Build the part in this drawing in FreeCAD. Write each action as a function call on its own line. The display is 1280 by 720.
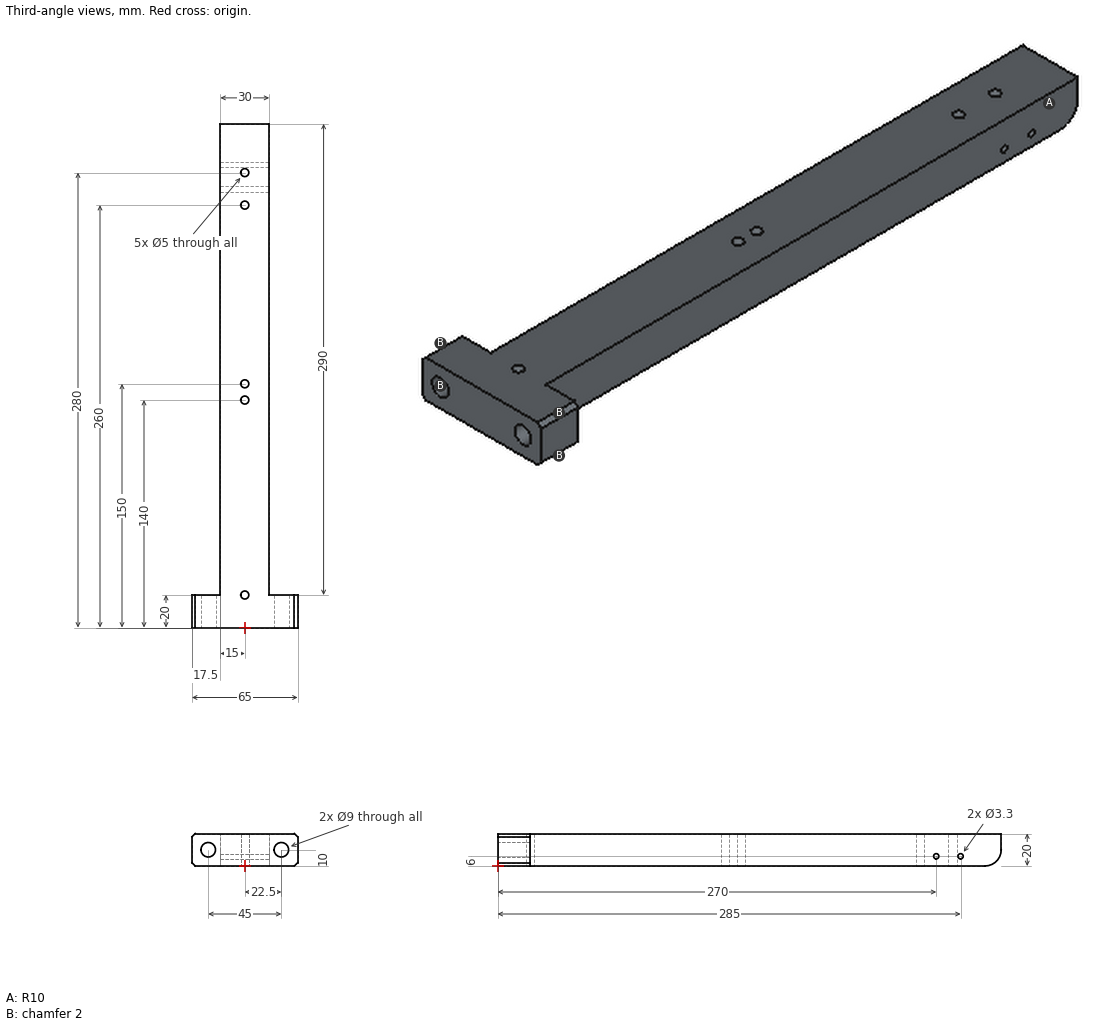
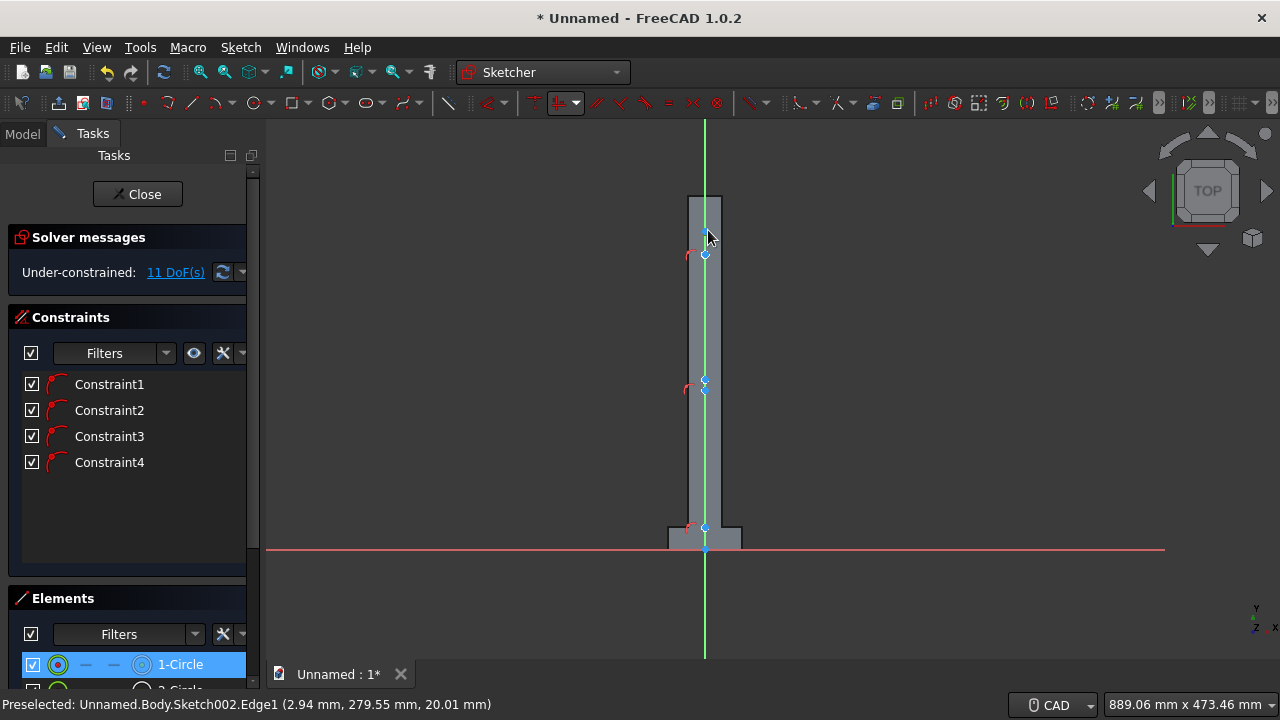
scroll(707, 378, up, 10)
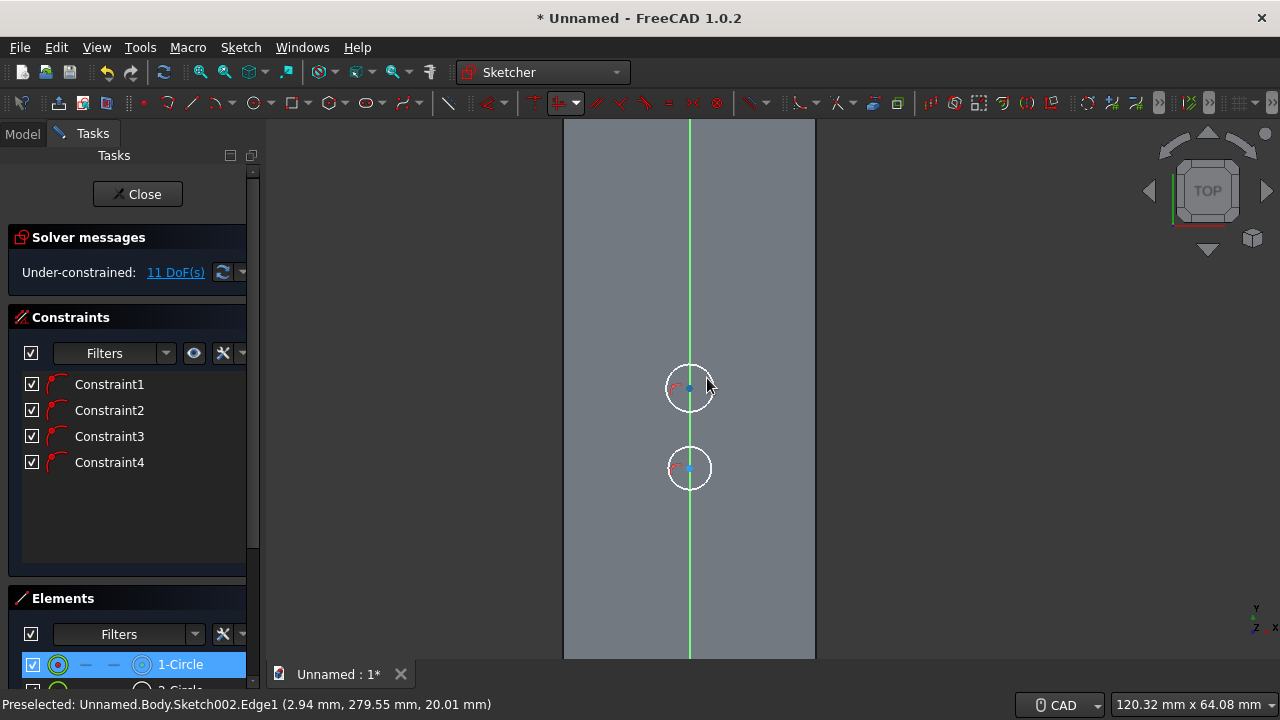
click(707, 371)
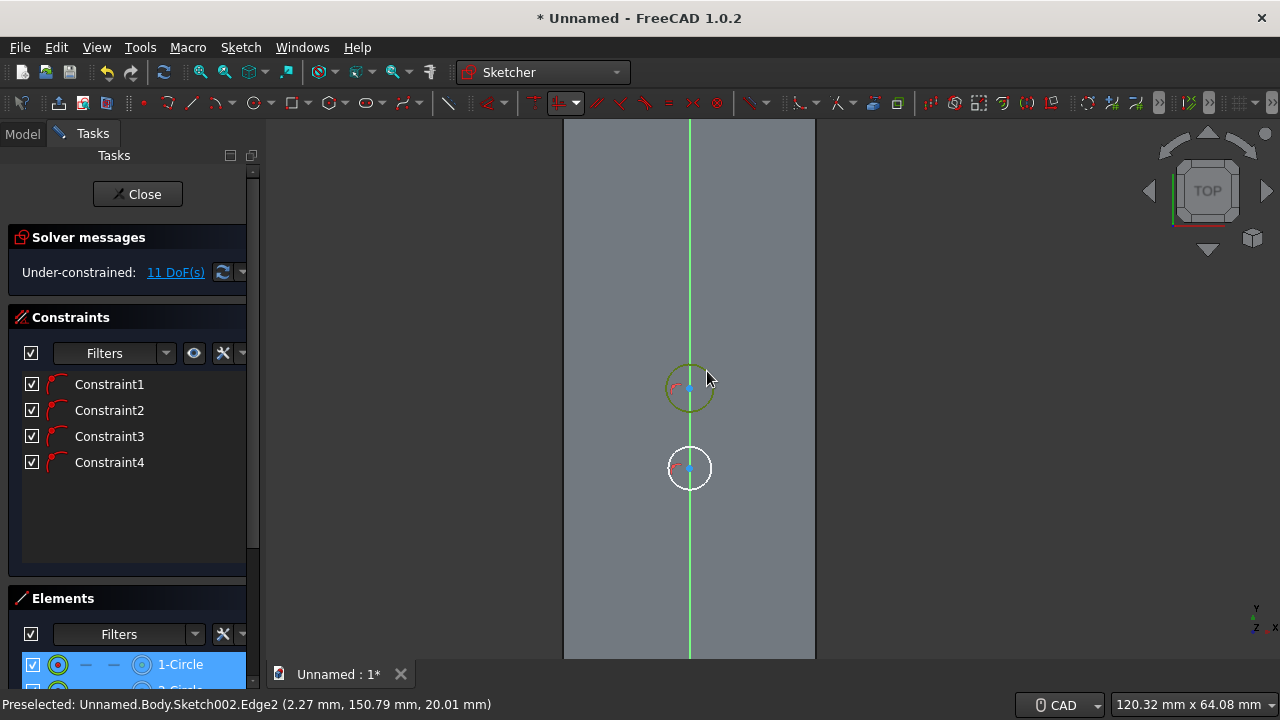
scroll(707, 379, down, 10)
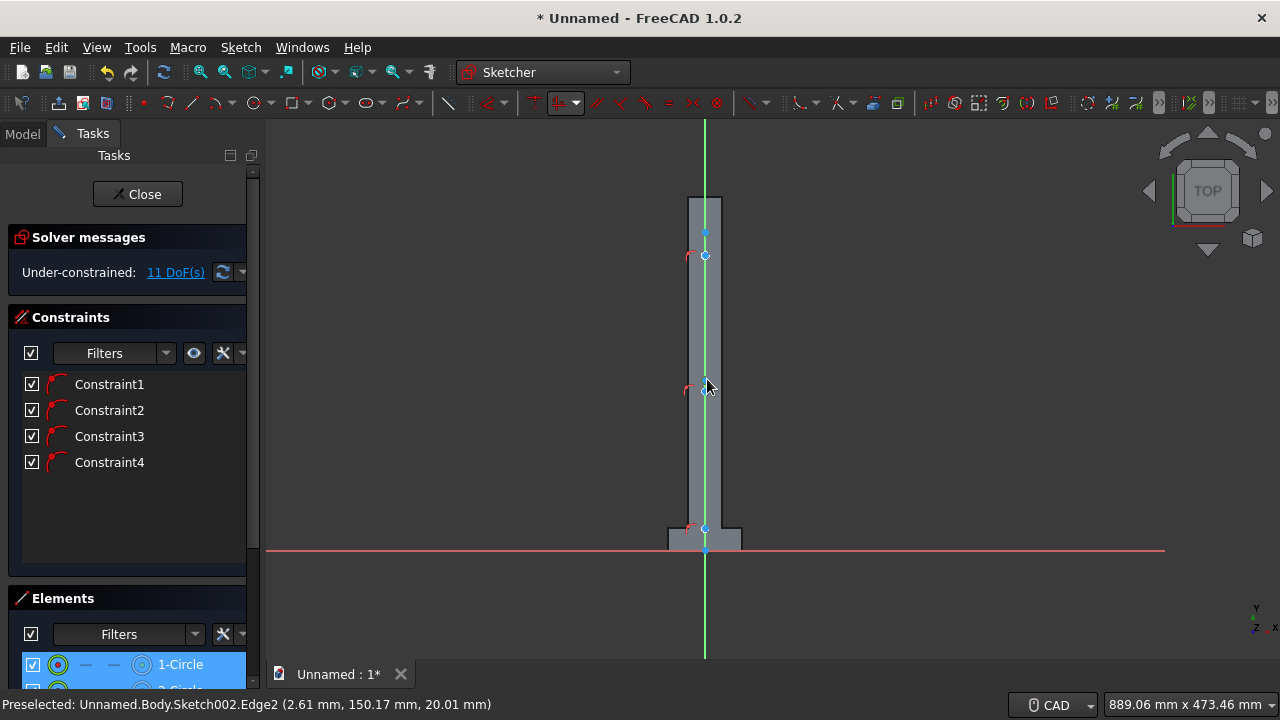
scroll(707, 527, up, 10)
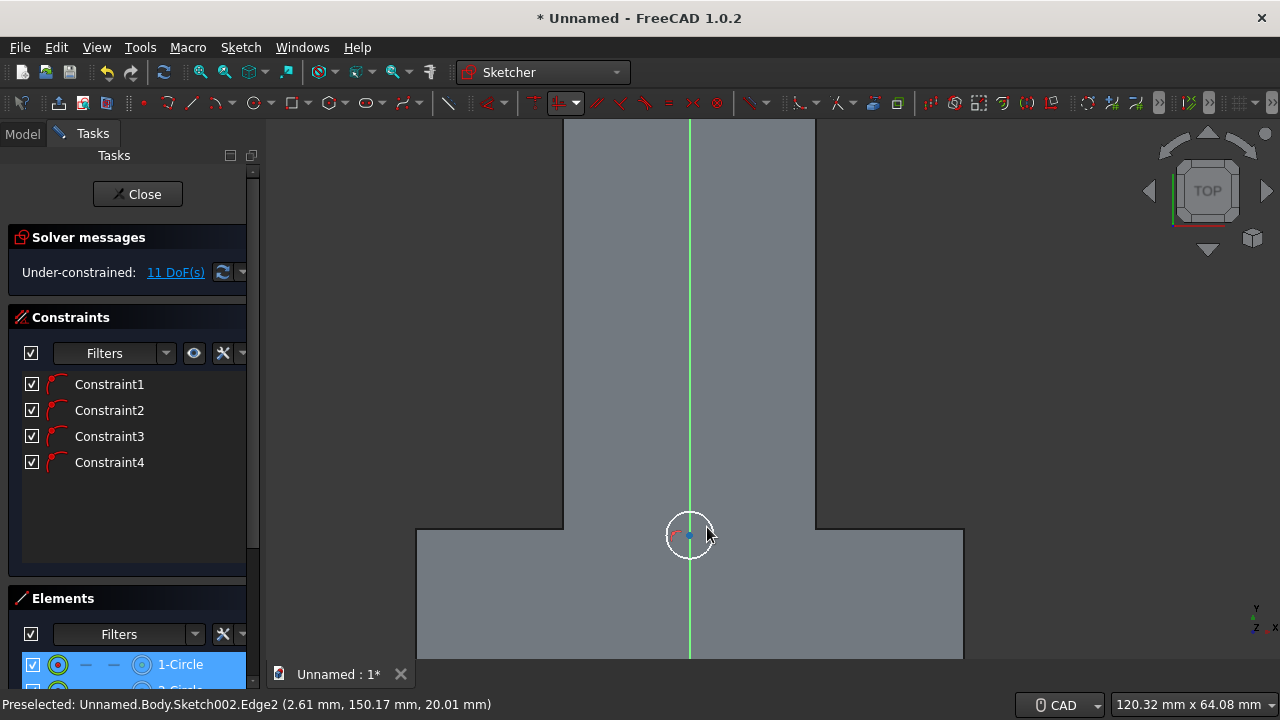
click(706, 519)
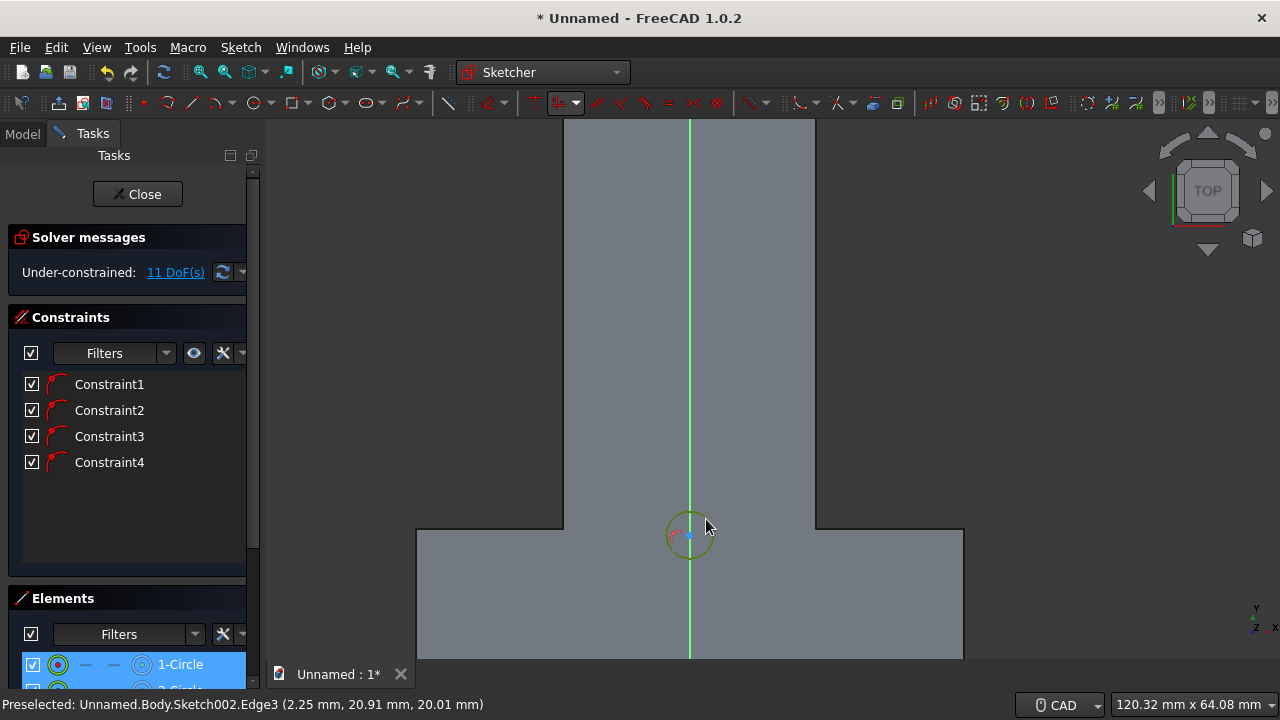
scroll(707, 527, down, 10)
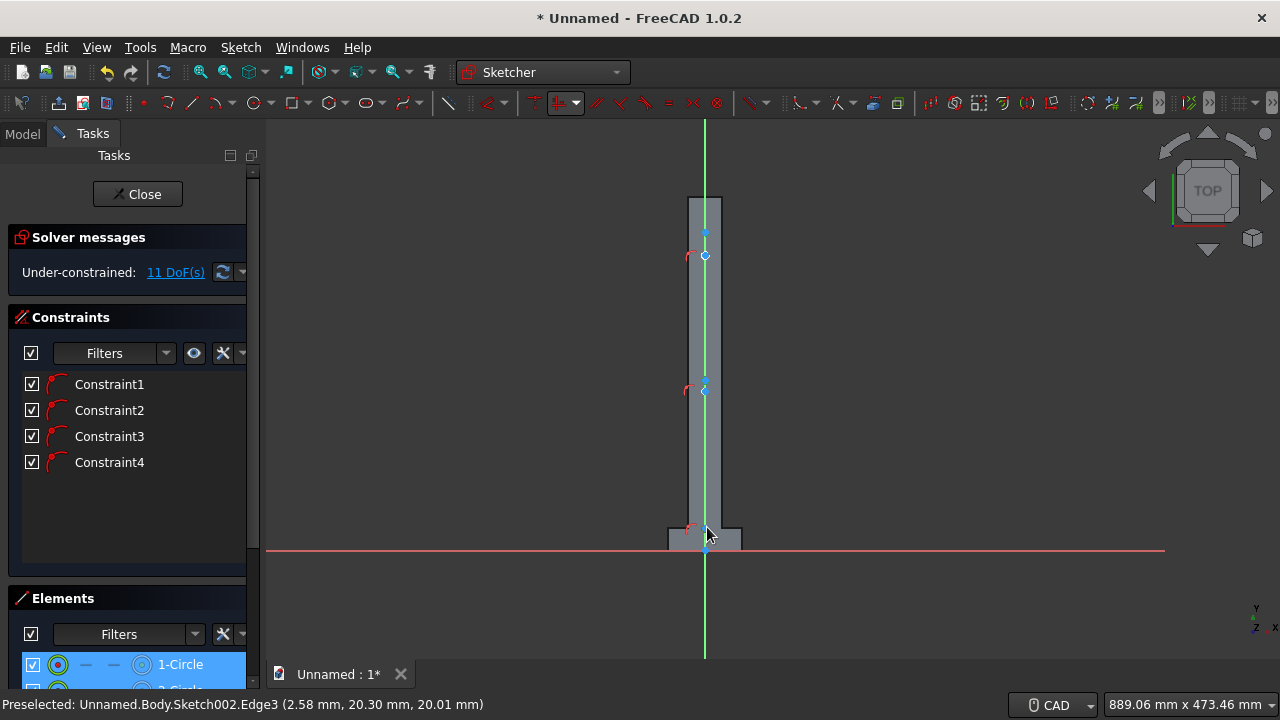
scroll(708, 253, up, 9)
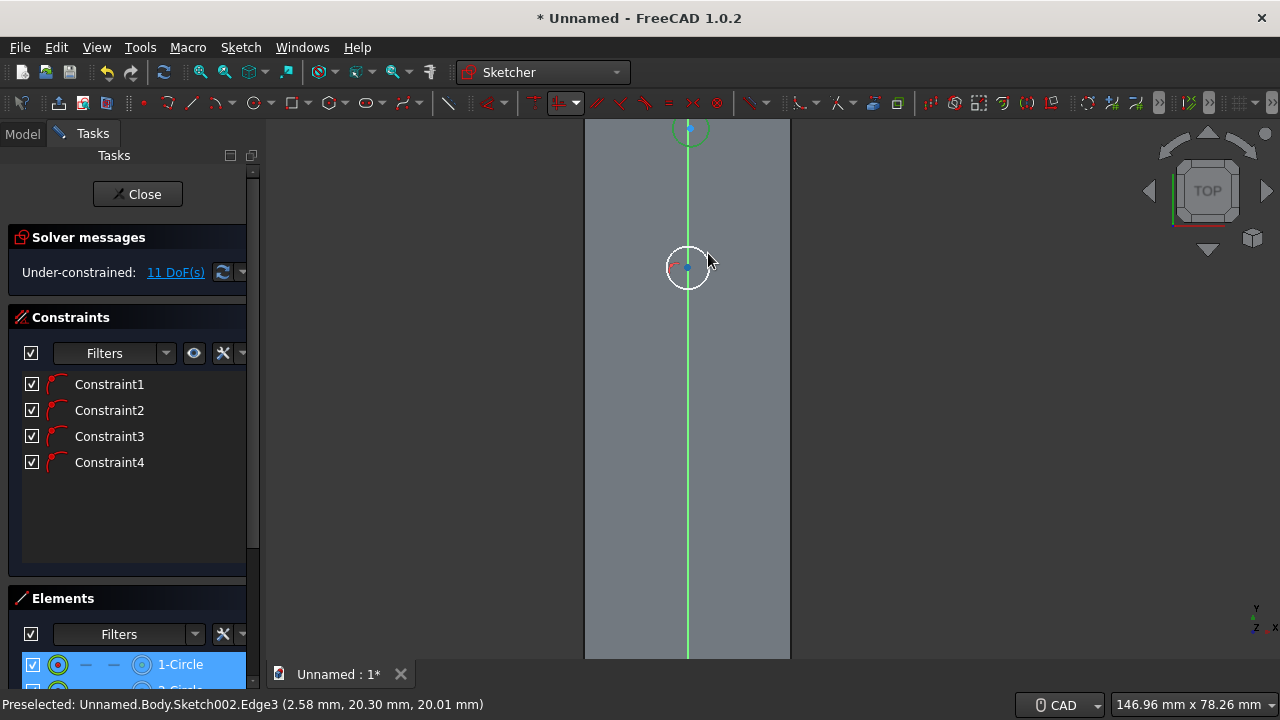
click(703, 253)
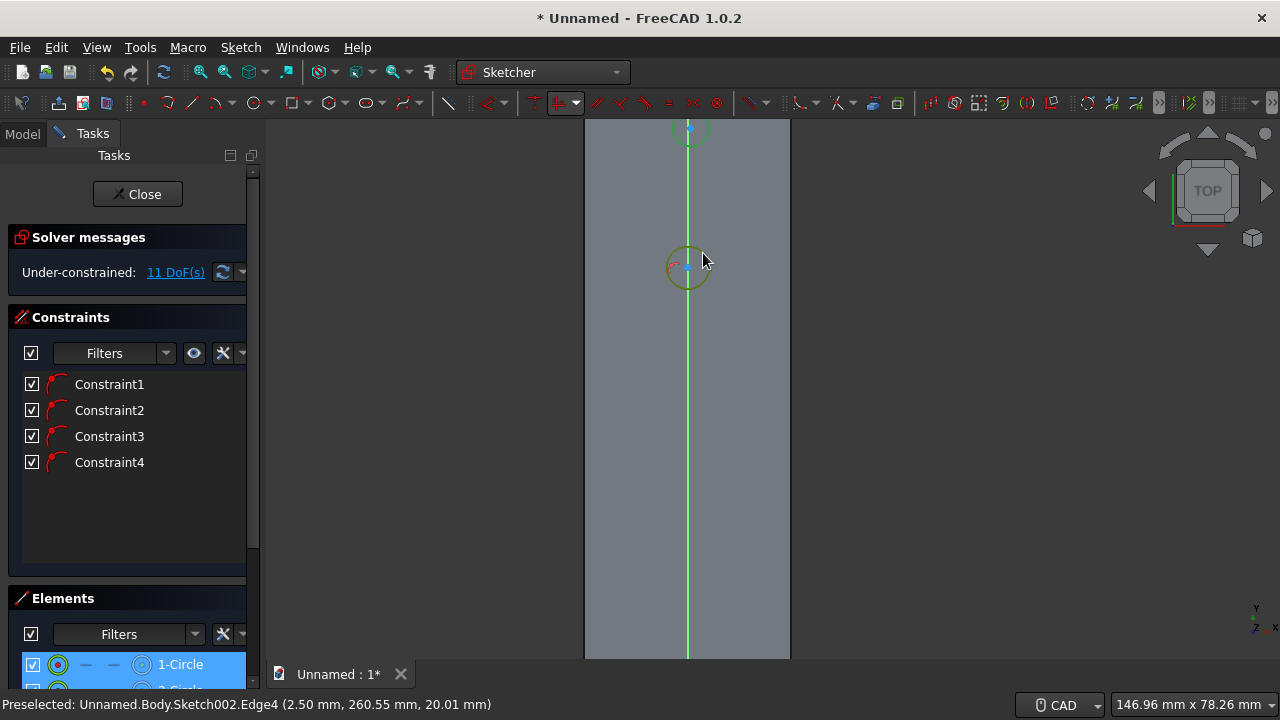
scroll(708, 252, down, 9)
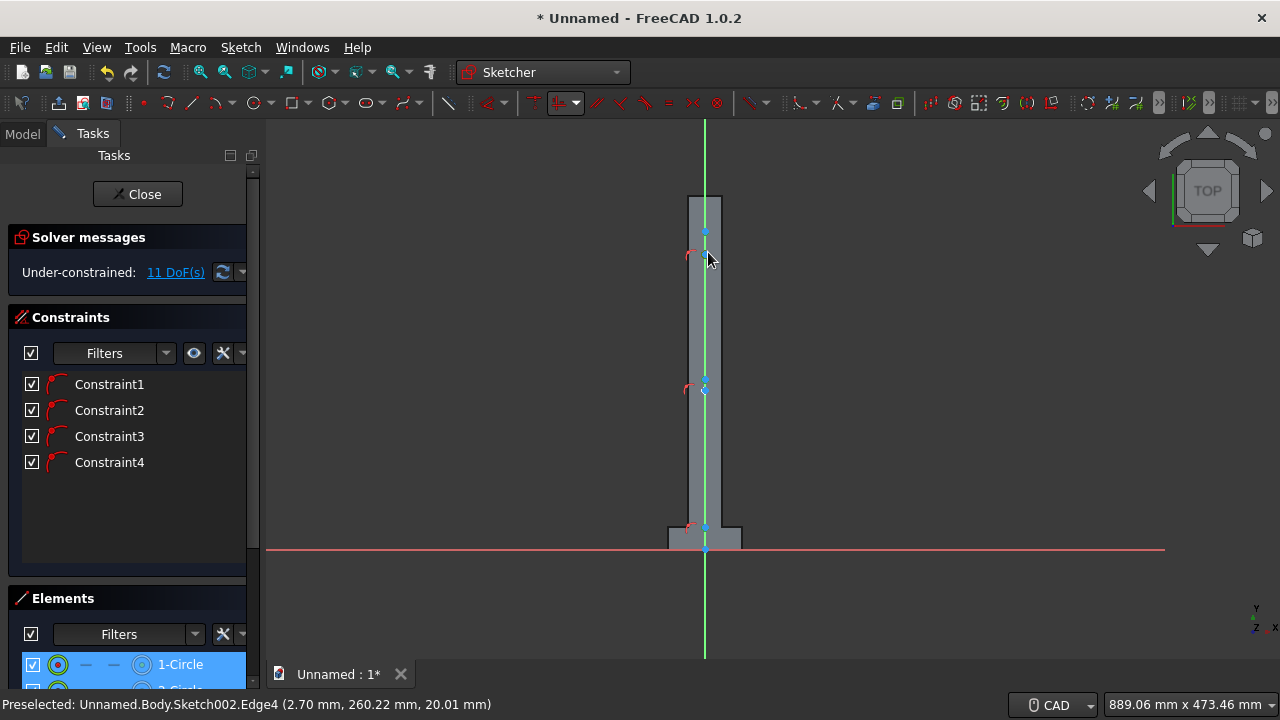
scroll(707, 389, up, 10)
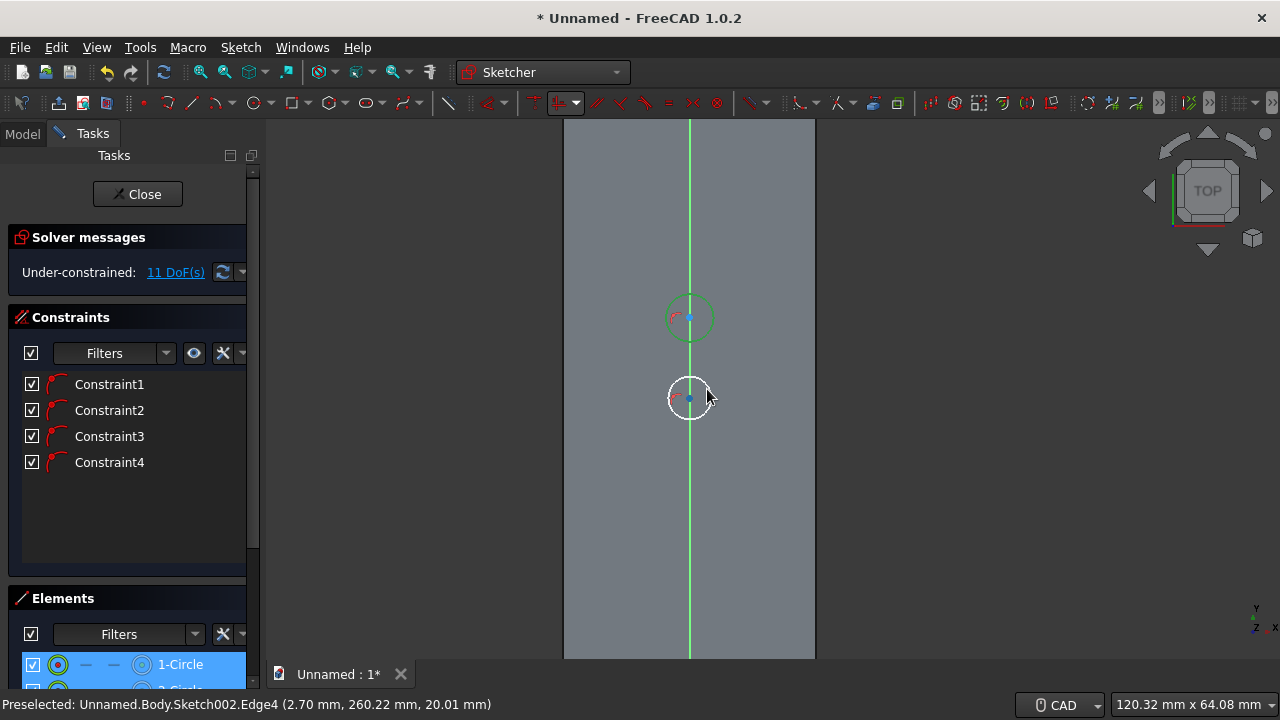
click(705, 383)